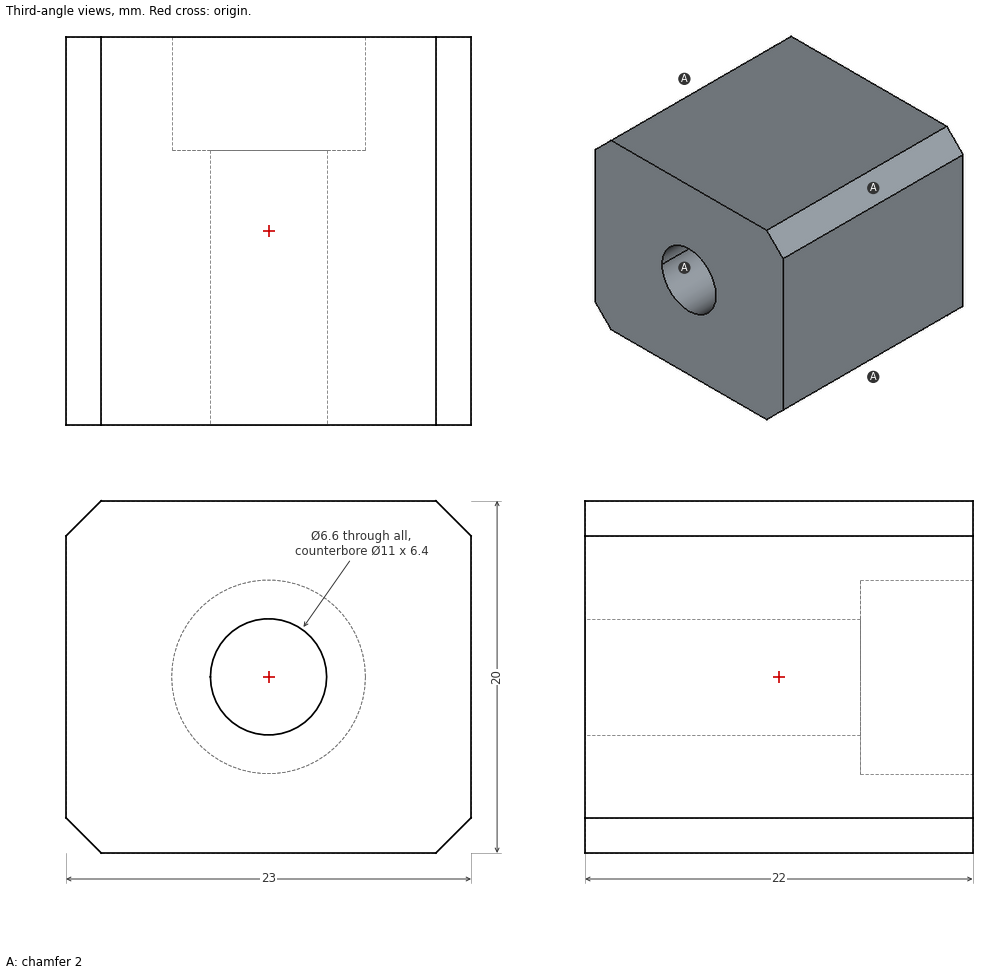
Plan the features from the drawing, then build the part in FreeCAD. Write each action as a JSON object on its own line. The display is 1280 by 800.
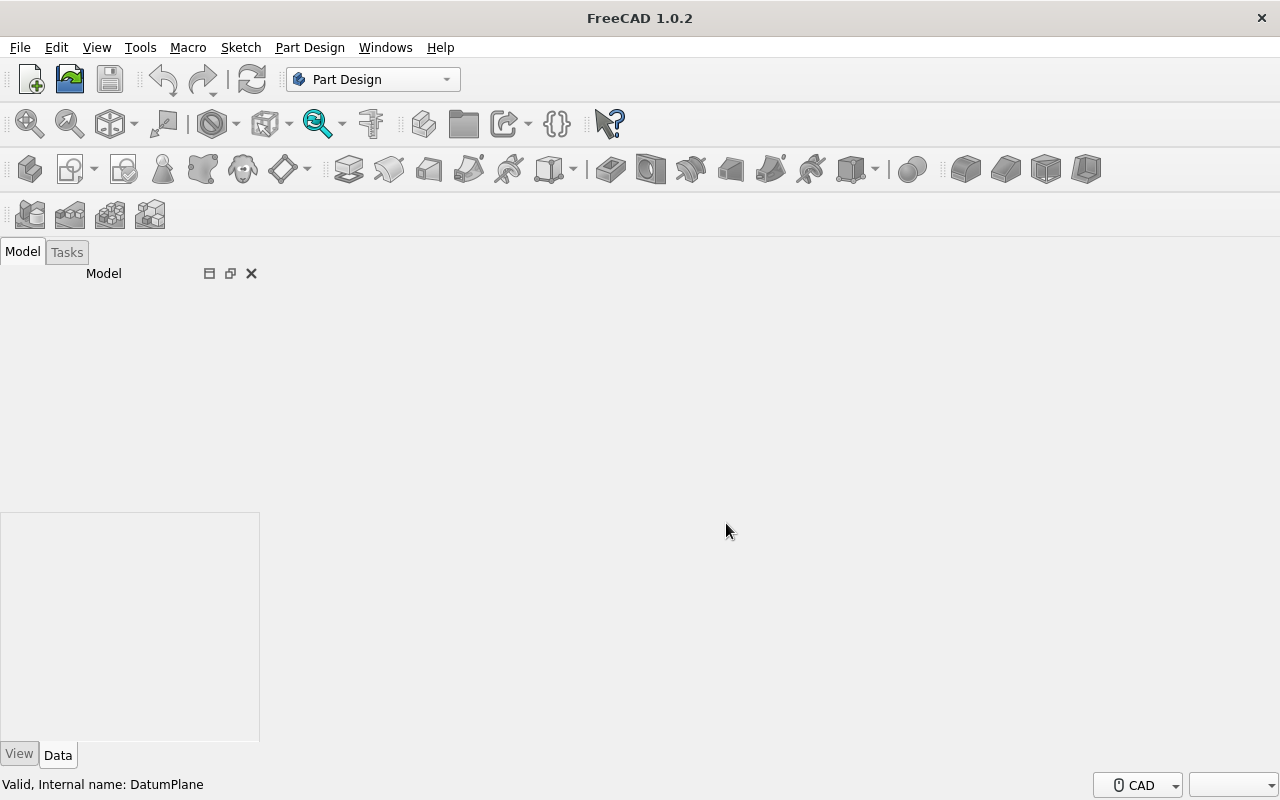
{"action": "left_click", "coordinate": [30, 80]}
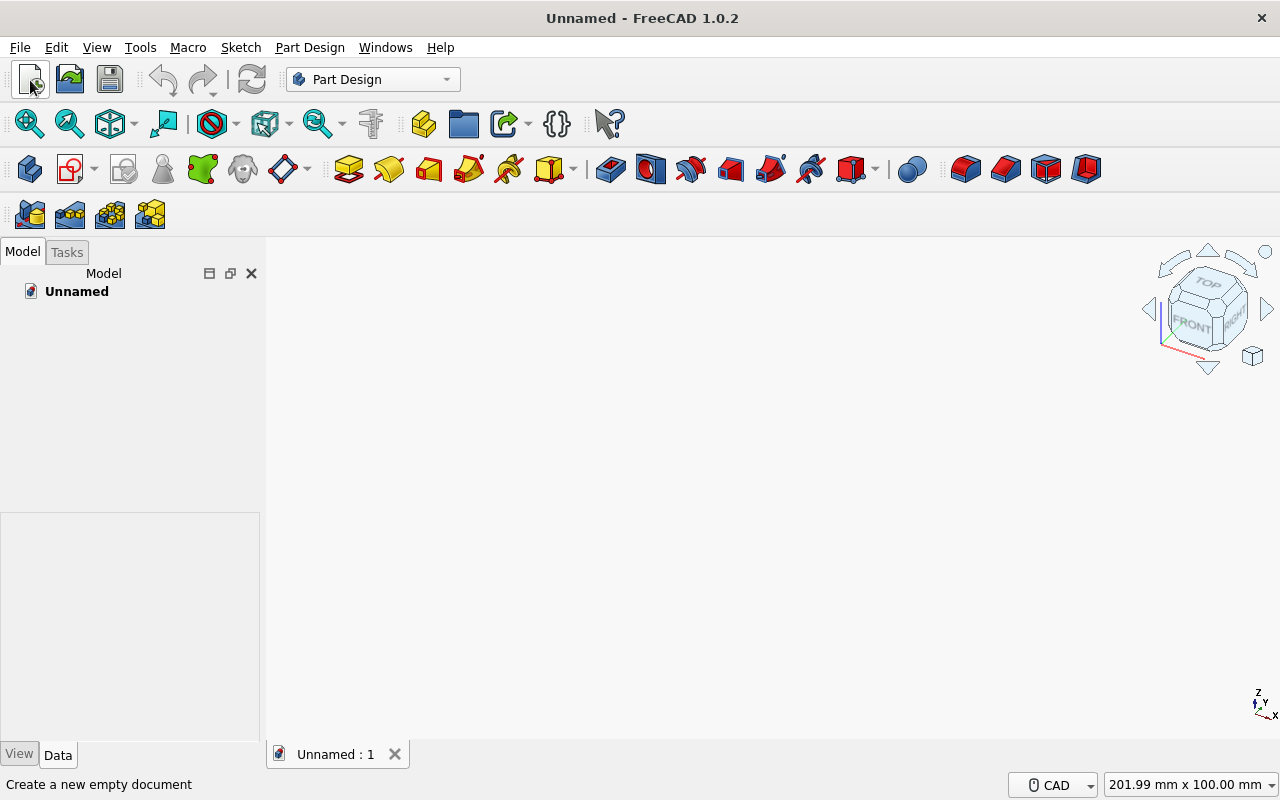
{"action": "left_click", "coordinate": [70, 170]}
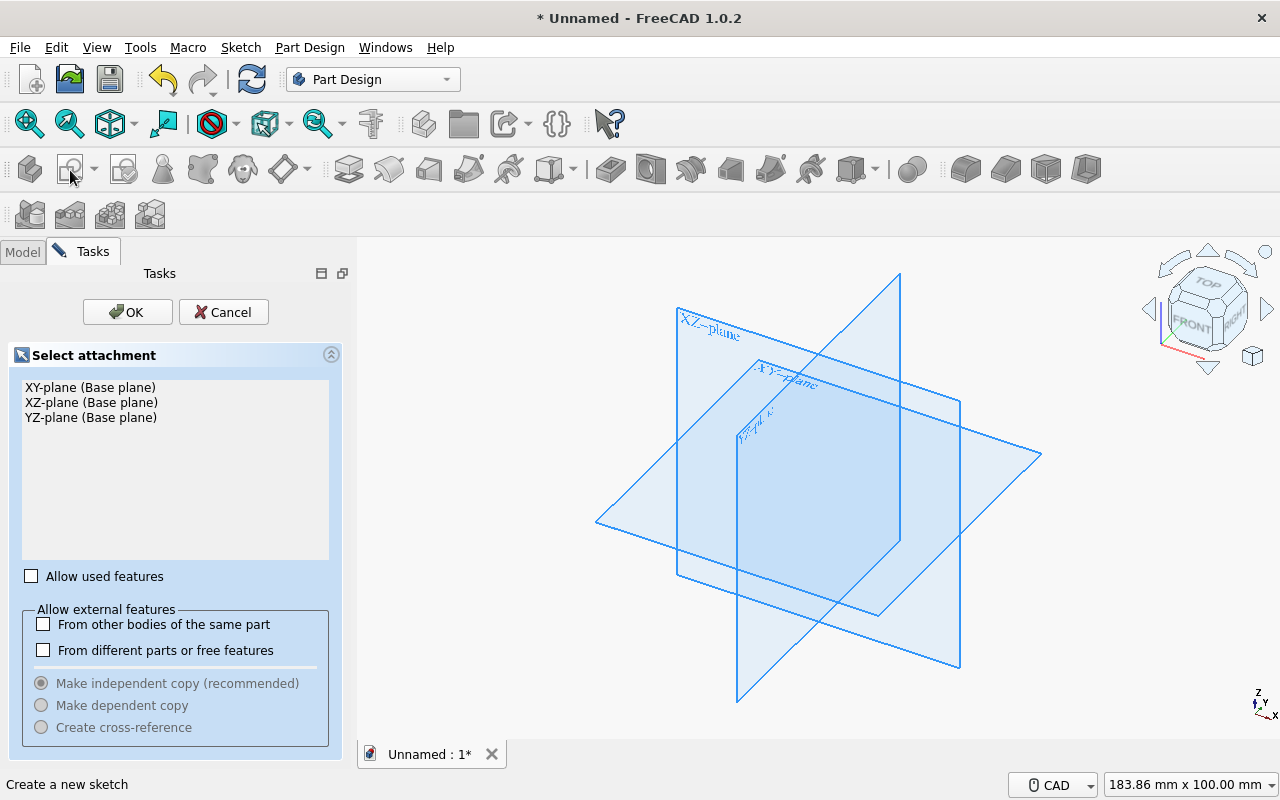
{"action": "left_click", "coordinate": [82, 402]}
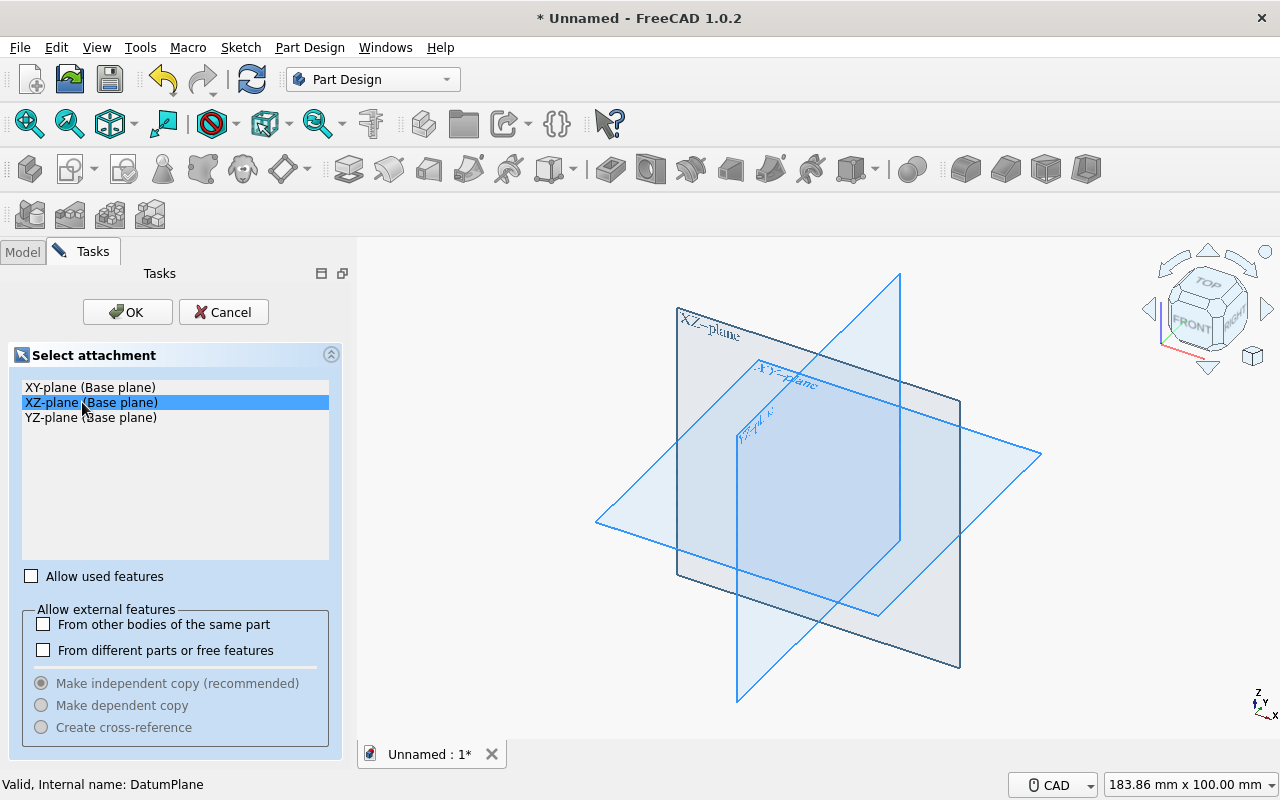
{"action": "left_click", "coordinate": [128, 312]}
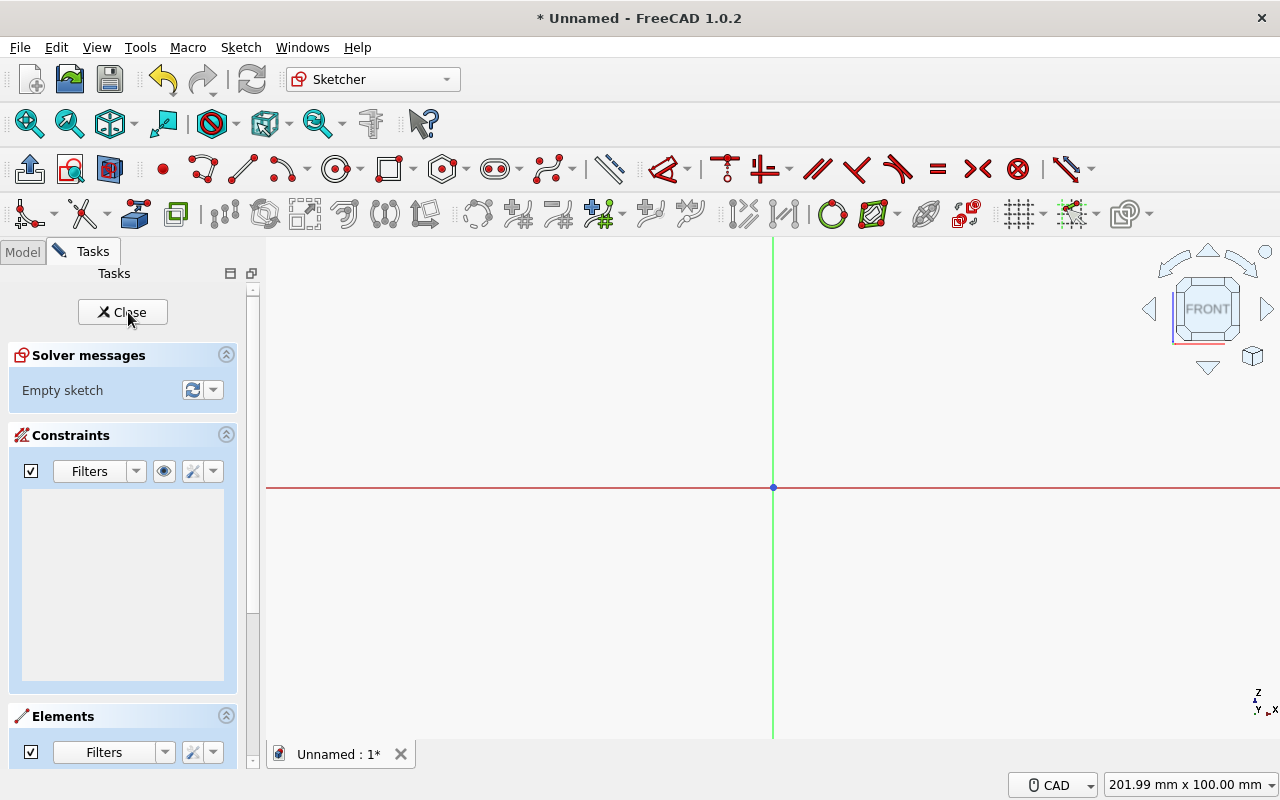
{"action": "scroll", "coordinate": [803, 488], "scroll_direction": "up", "scroll_amount": 6}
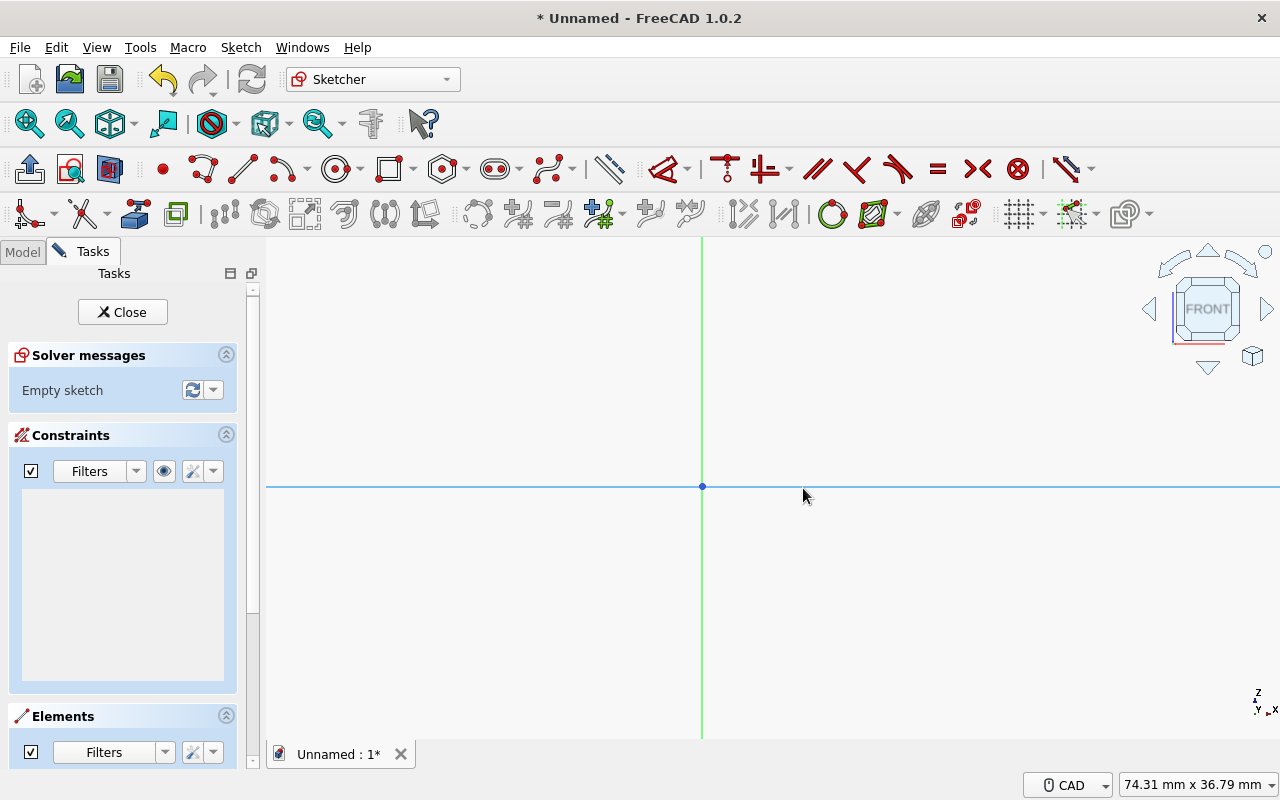
{"action": "key", "text": "g v"}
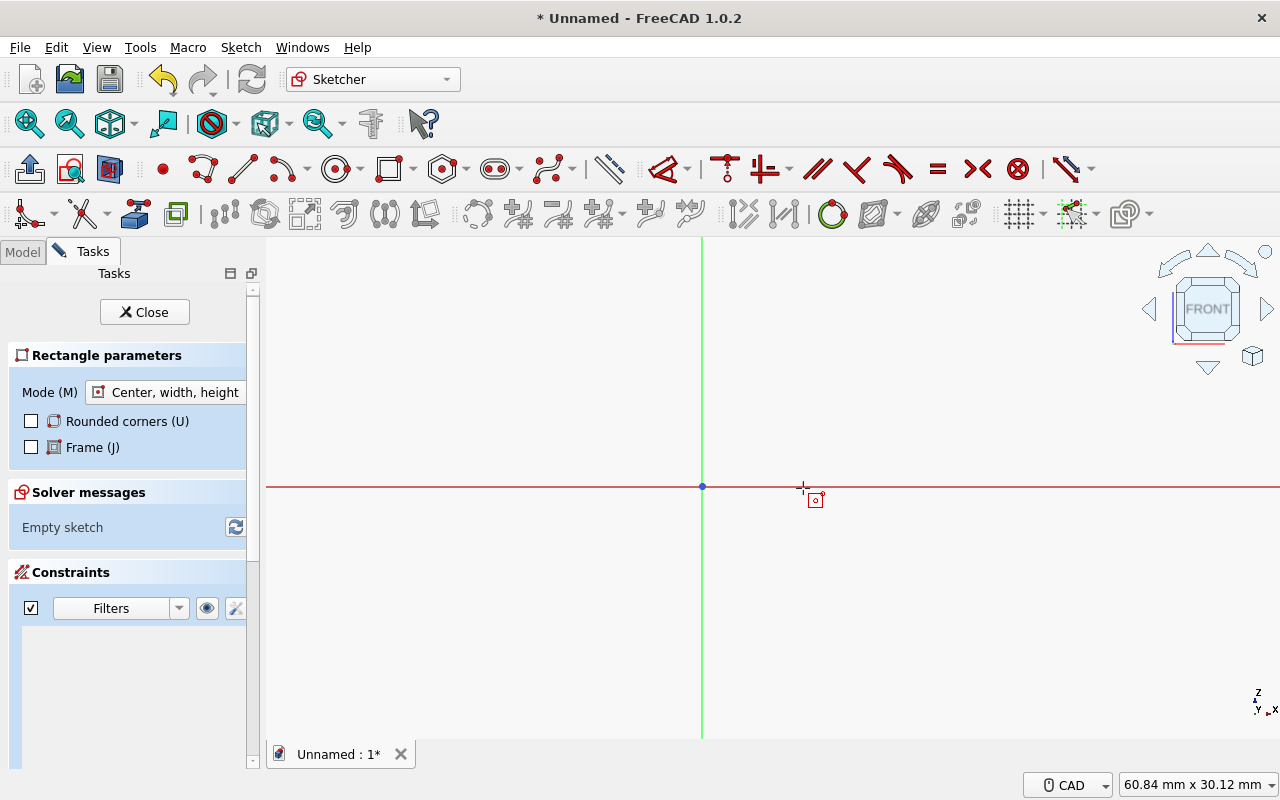
{"action": "left_click", "coordinate": [702, 487]}
{"action": "mouse_move", "coordinate": [894, 320]}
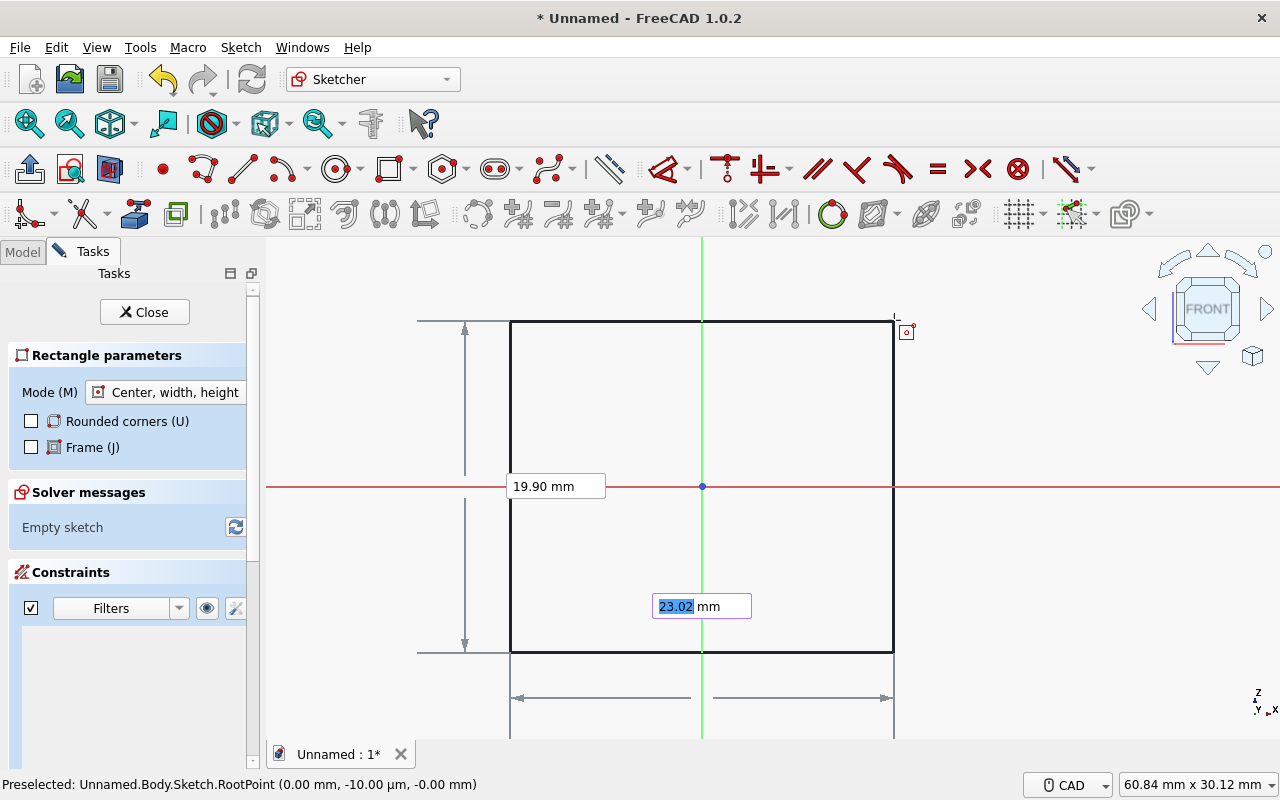
{"action": "type", "text": "23"}
{"action": "key", "text": "Tab"}
{"action": "type", "text": "20"}
{"action": "key", "text": "Return"}
{"action": "key", "text": "Escape"}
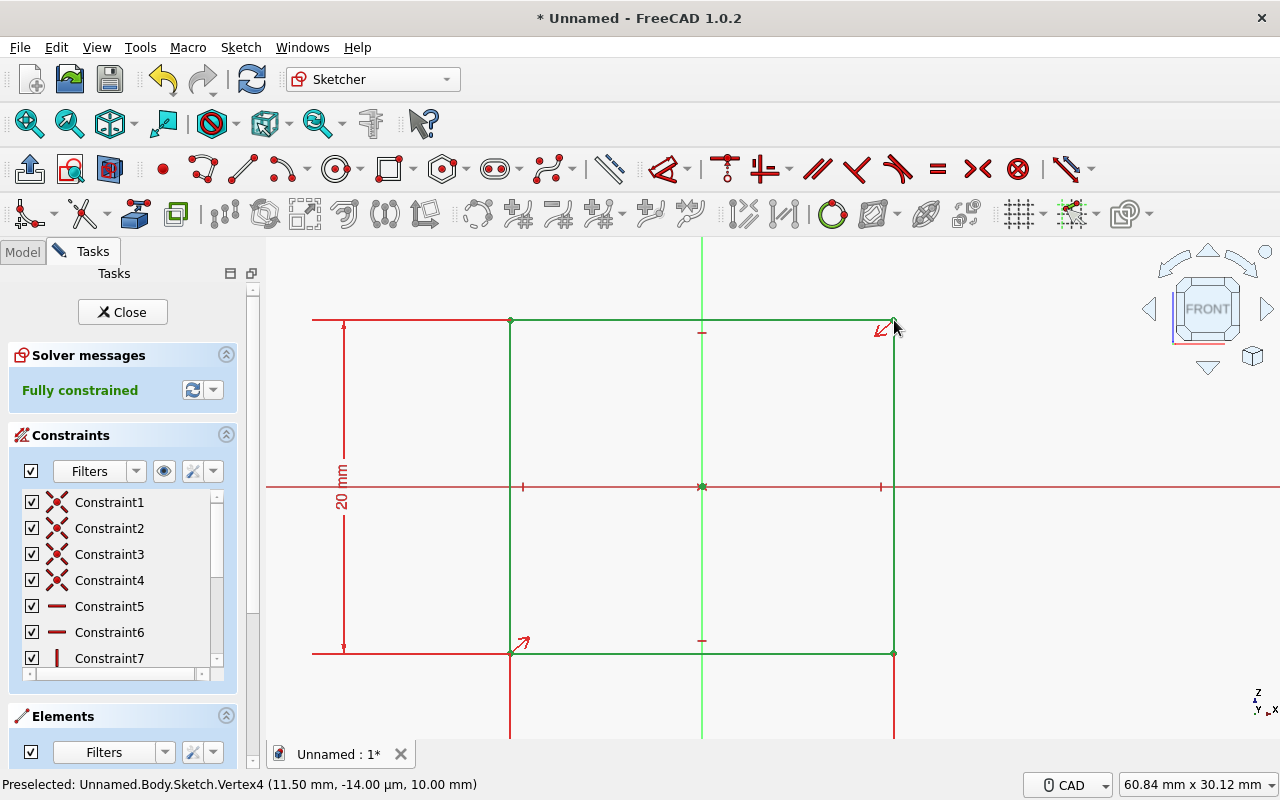
{"action": "left_click", "coordinate": [123, 312]}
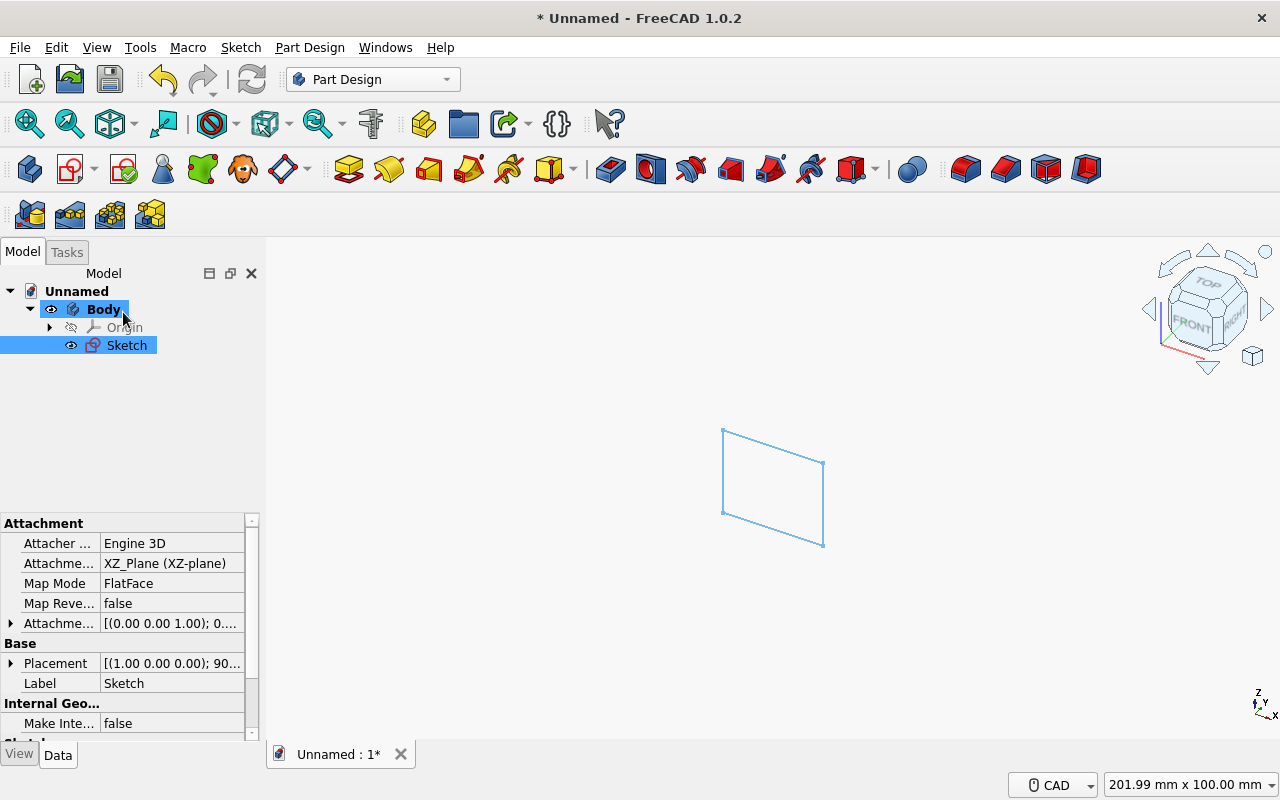
{"action": "left_click", "coordinate": [350, 170]}